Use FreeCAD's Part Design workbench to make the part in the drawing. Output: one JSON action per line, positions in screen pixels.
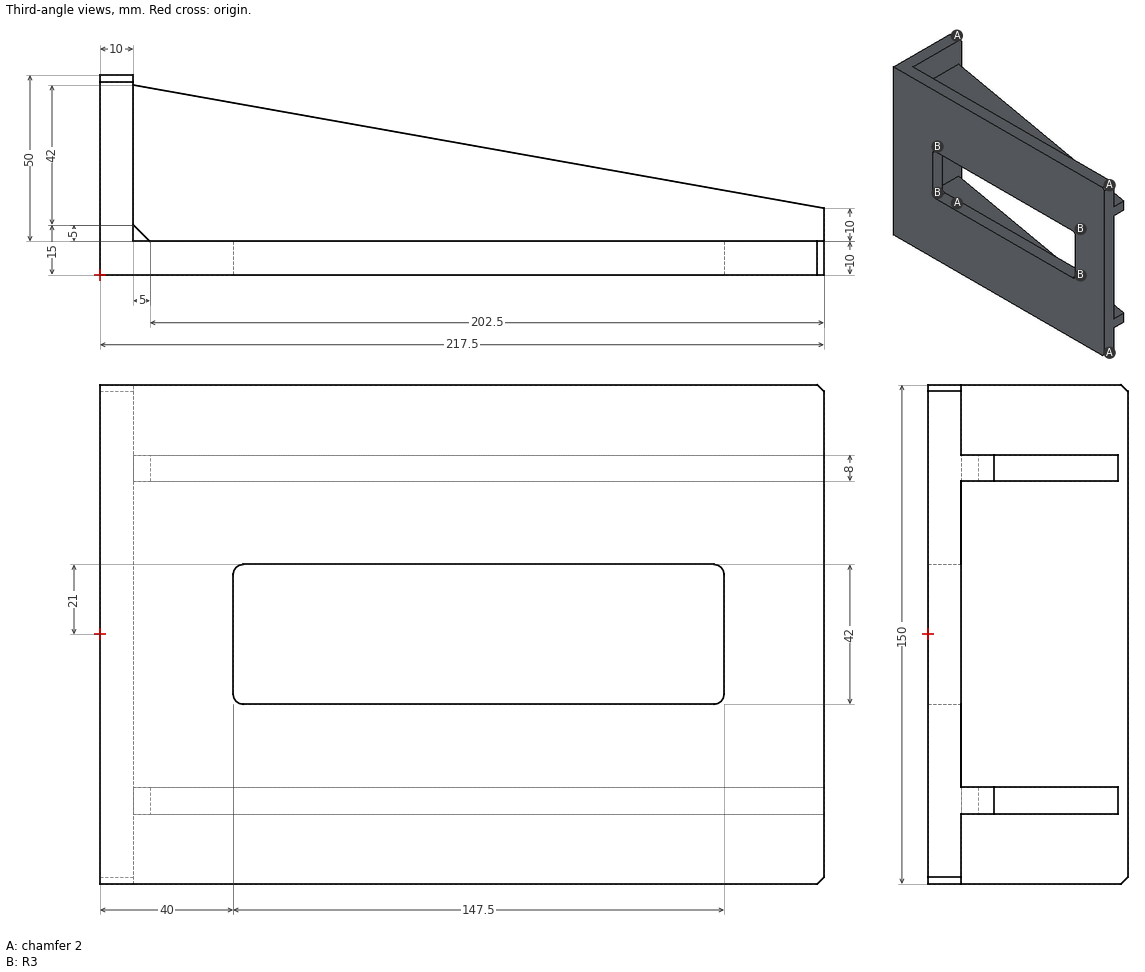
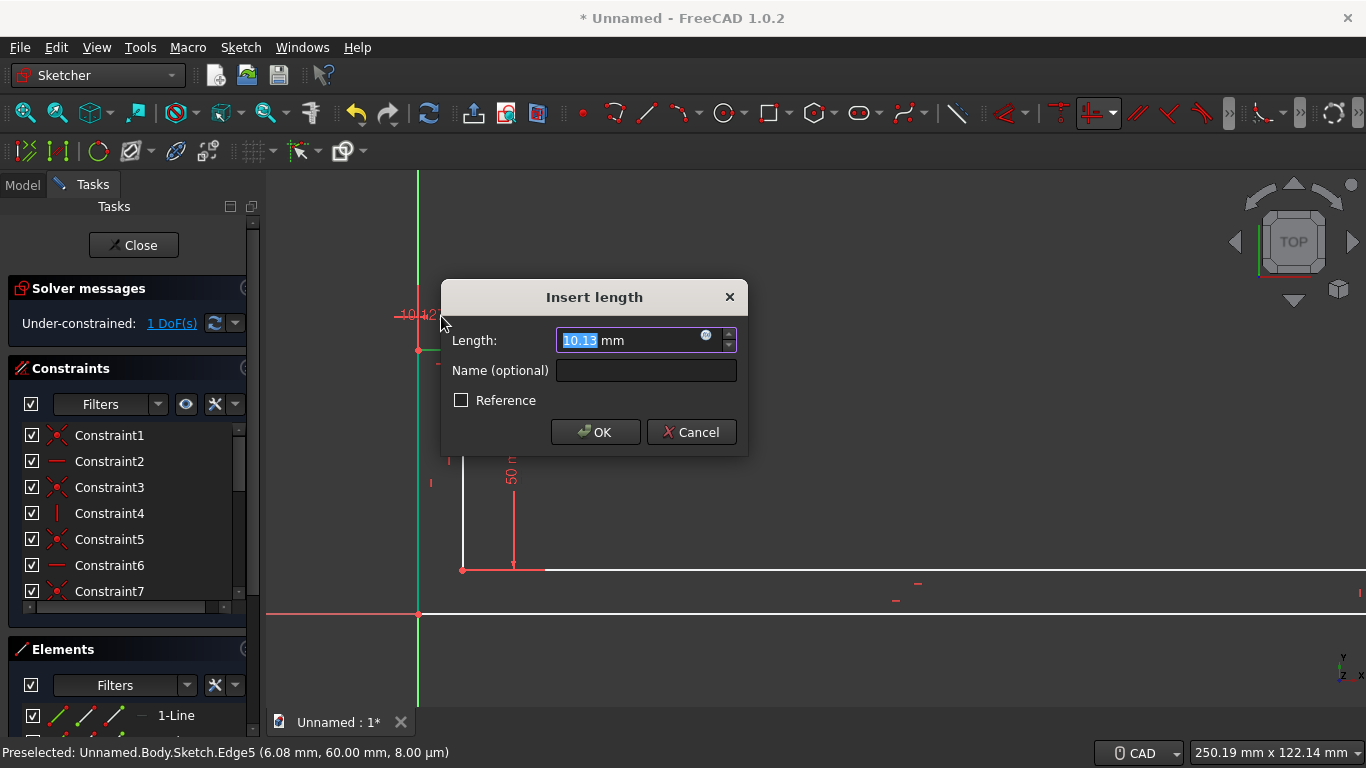
{"action": "type", "text": "10"}
{"action": "key", "text": "Return"}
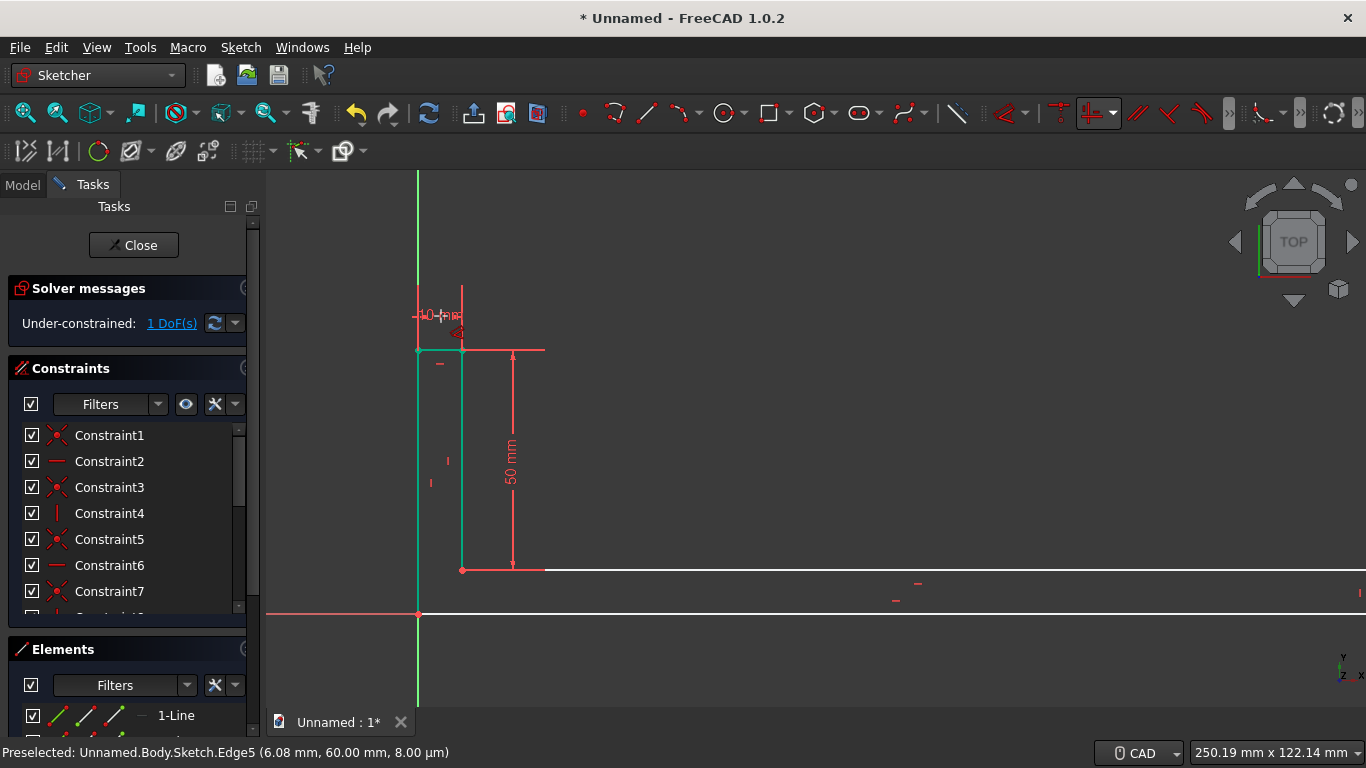
{"action": "left_click", "coordinate": [705, 614]}
{"action": "left_click", "coordinate": [810, 648]}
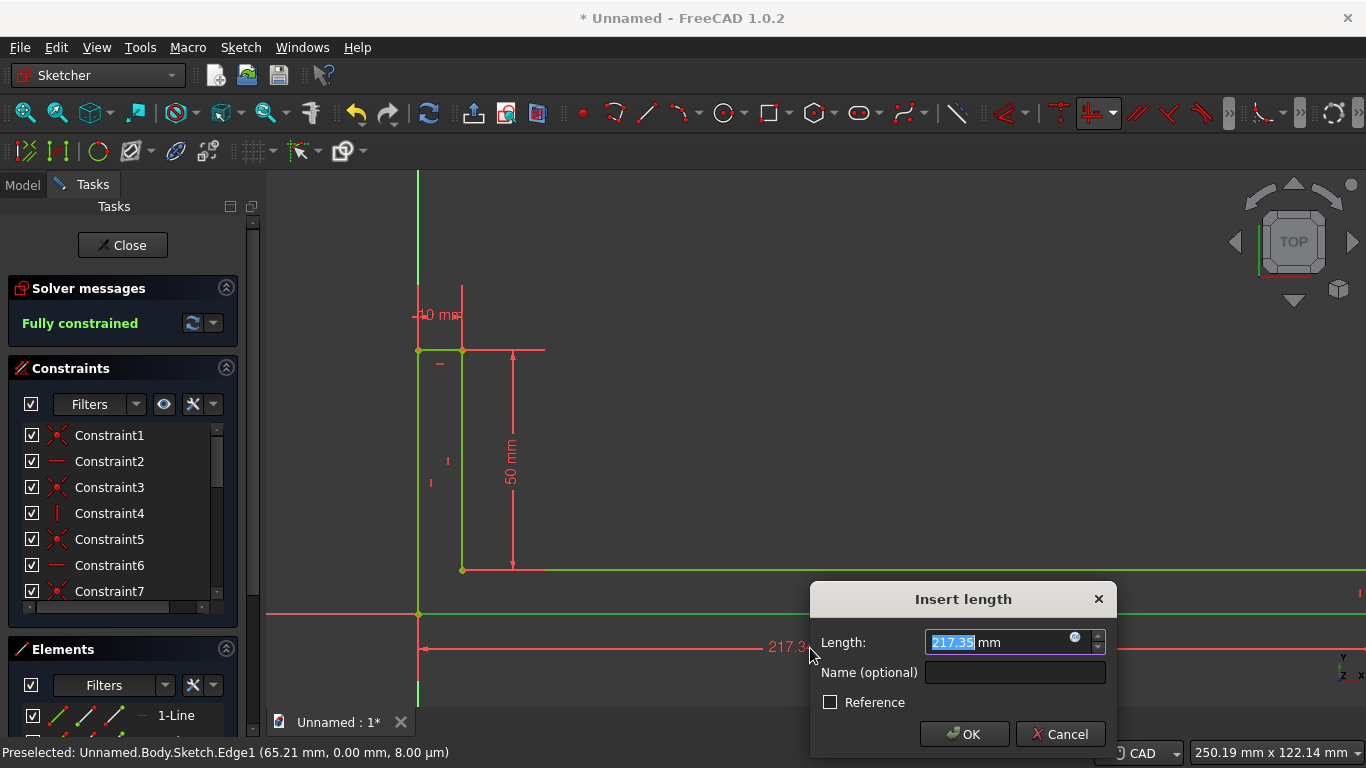
{"action": "type", "text": "217.5"}
{"action": "key", "text": "Return"}
{"action": "key", "text": "Escape"}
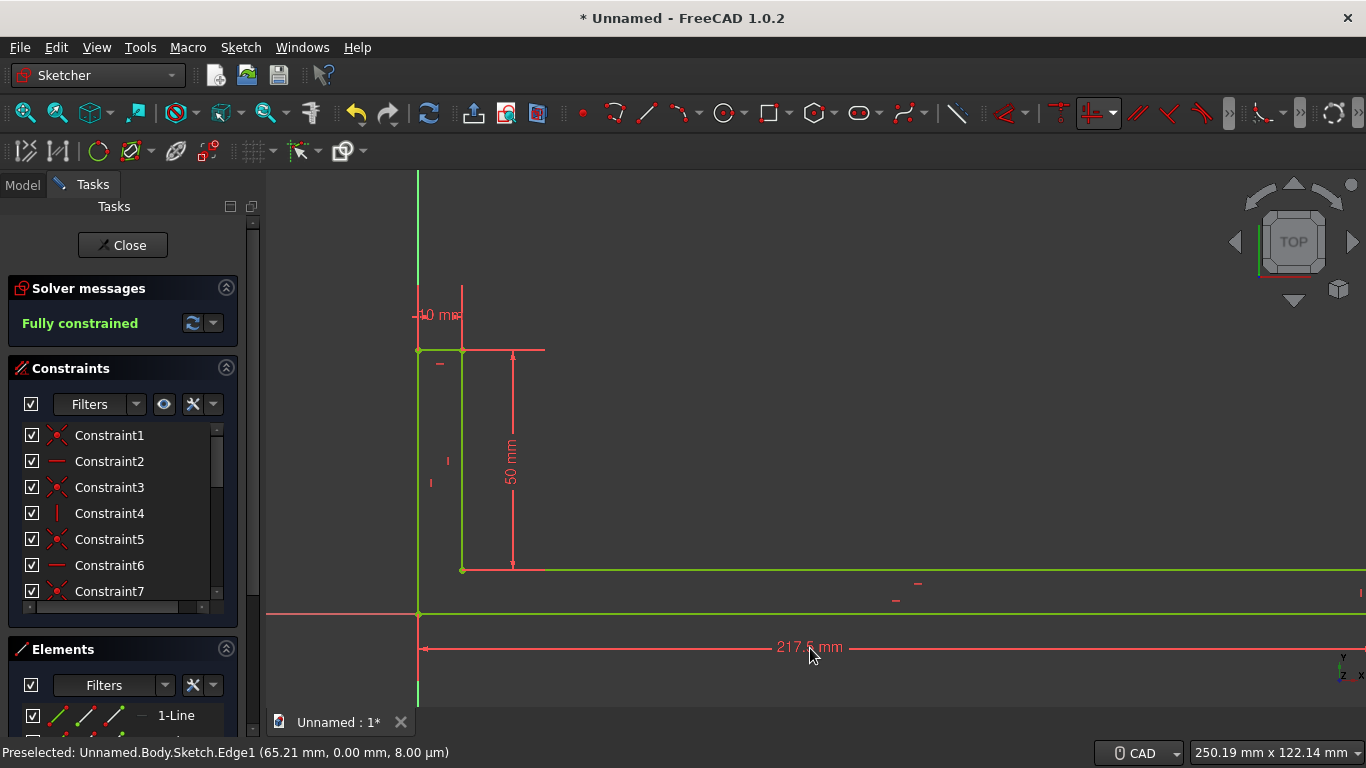
{"action": "left_click", "coordinate": [123, 245]}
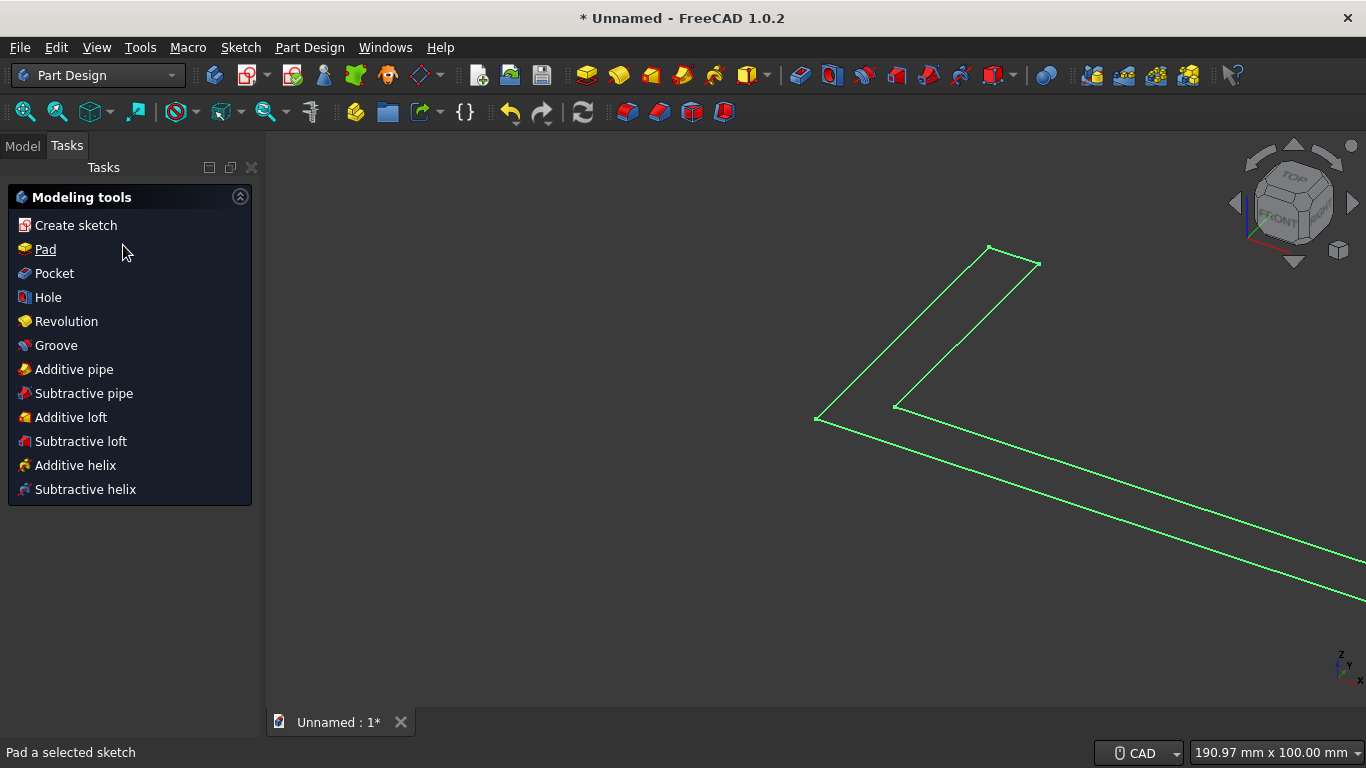
{"action": "left_click", "coordinate": [588, 76]}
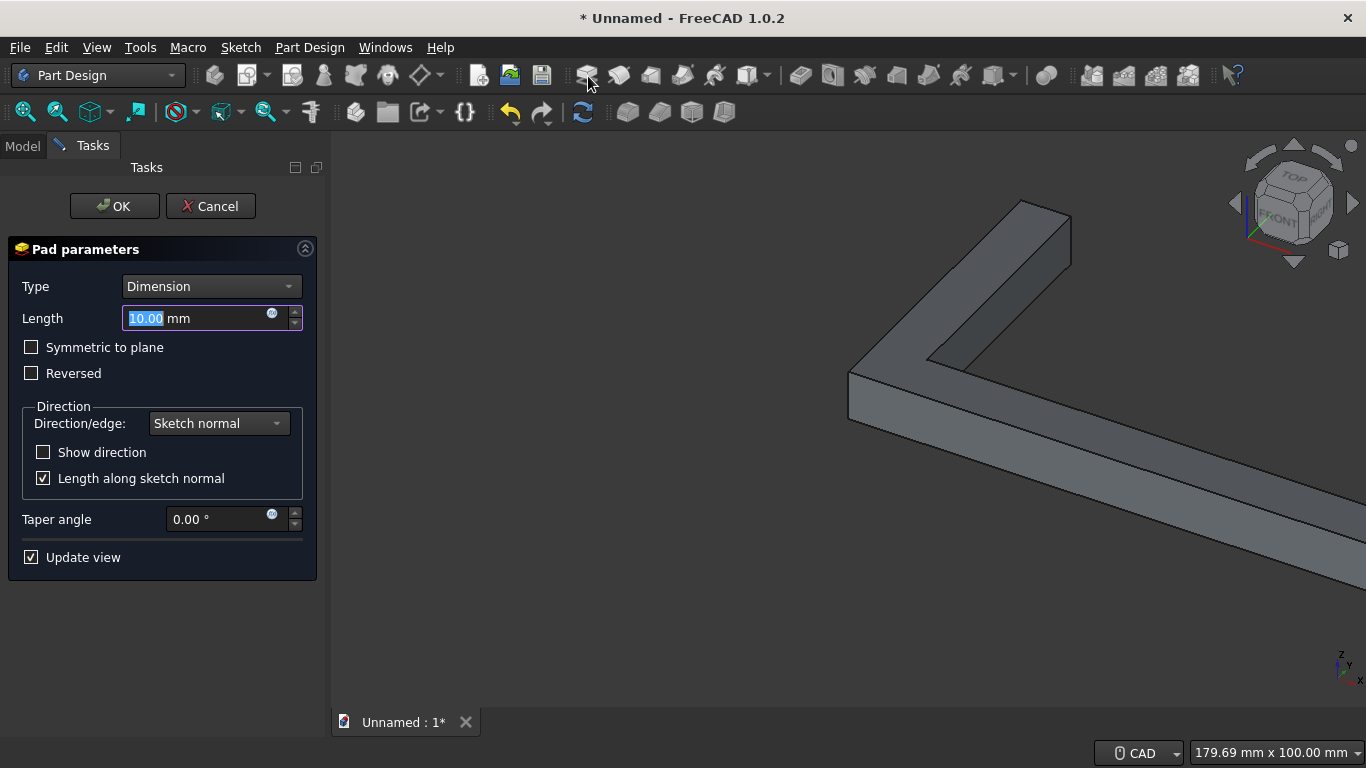
{"action": "type", "text": "150"}
{"action": "key", "text": "Tab"}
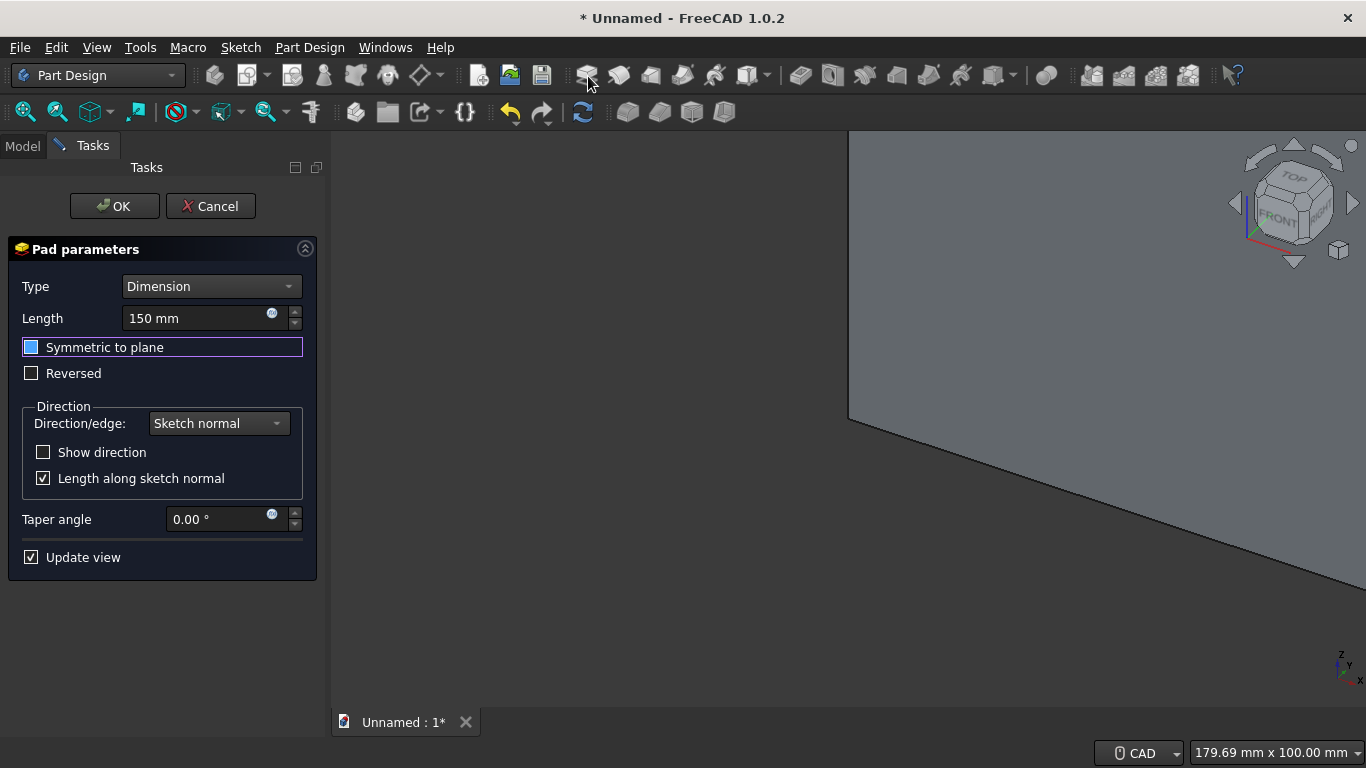
{"action": "left_click", "coordinate": [30, 347]}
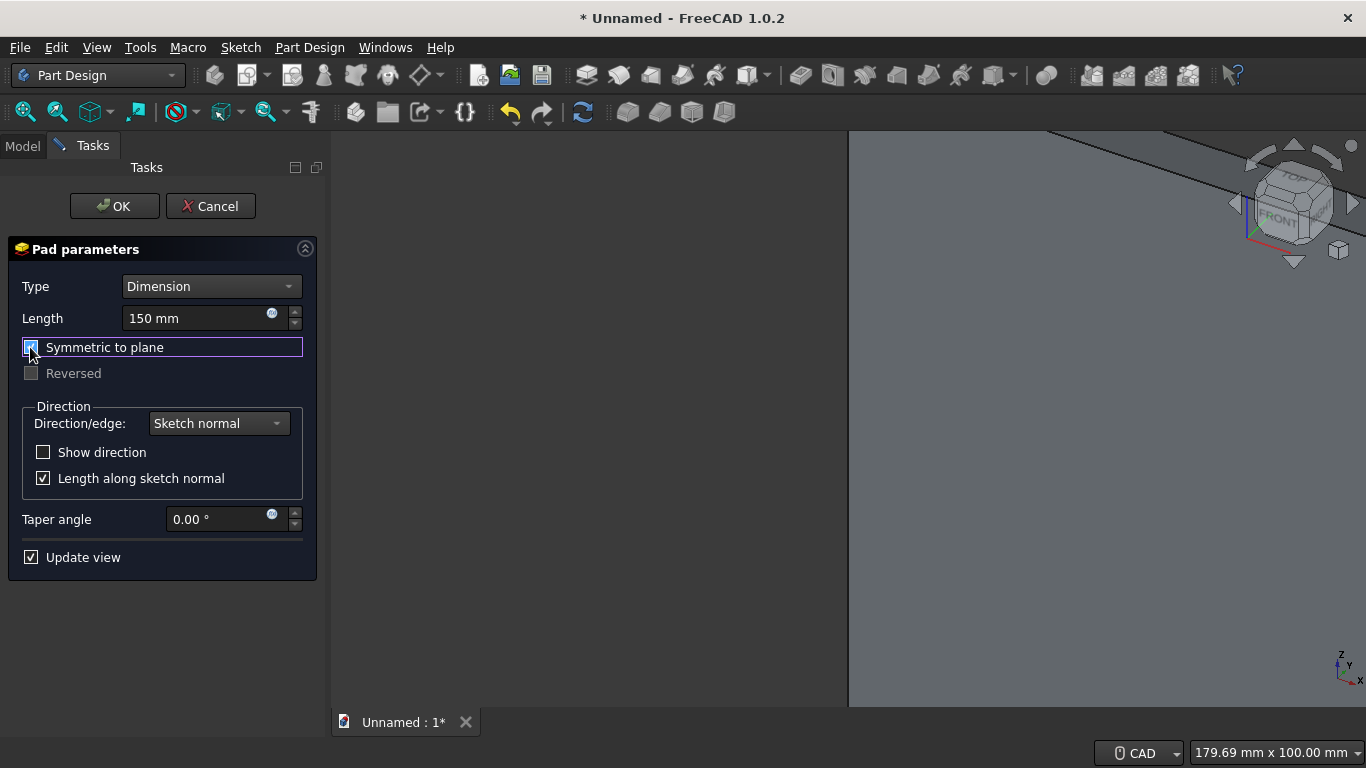
{"action": "left_click", "coordinate": [115, 206]}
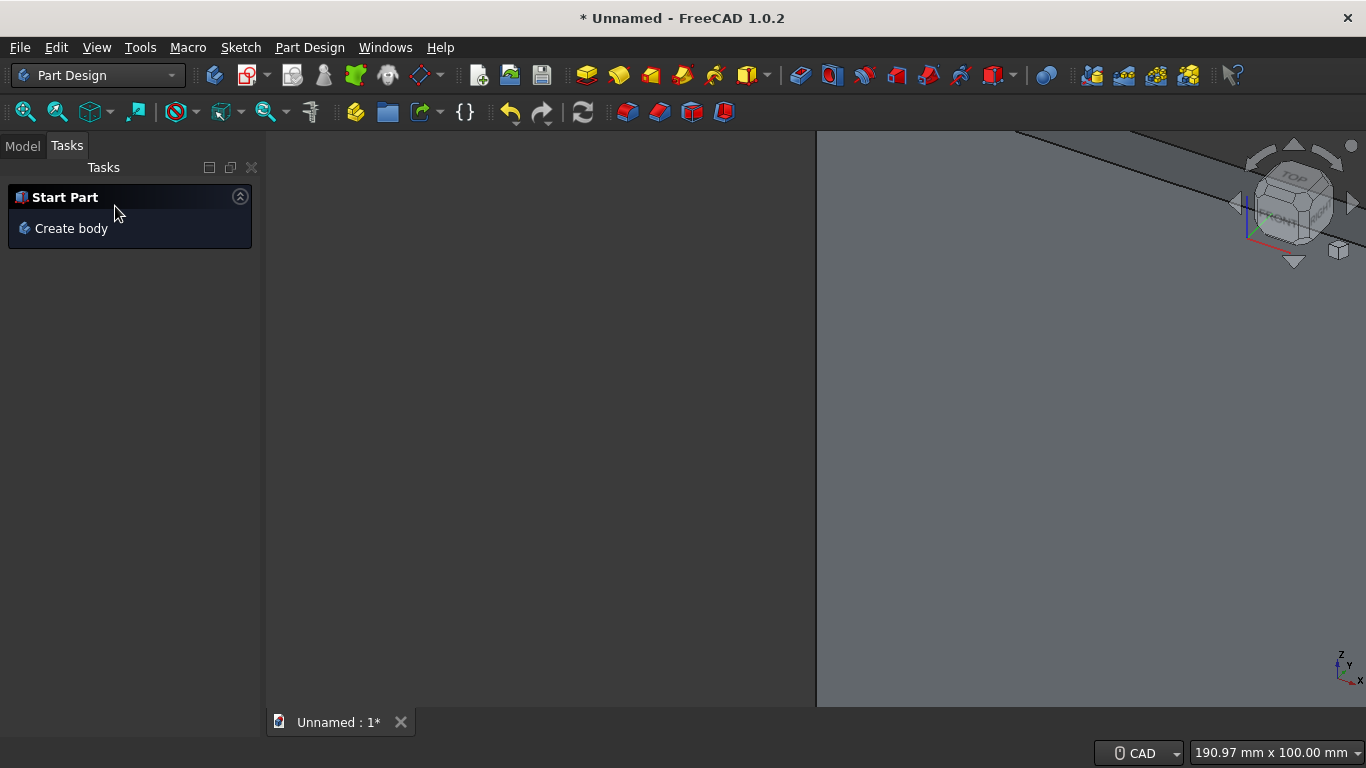
{"action": "left_click", "coordinate": [26, 112]}